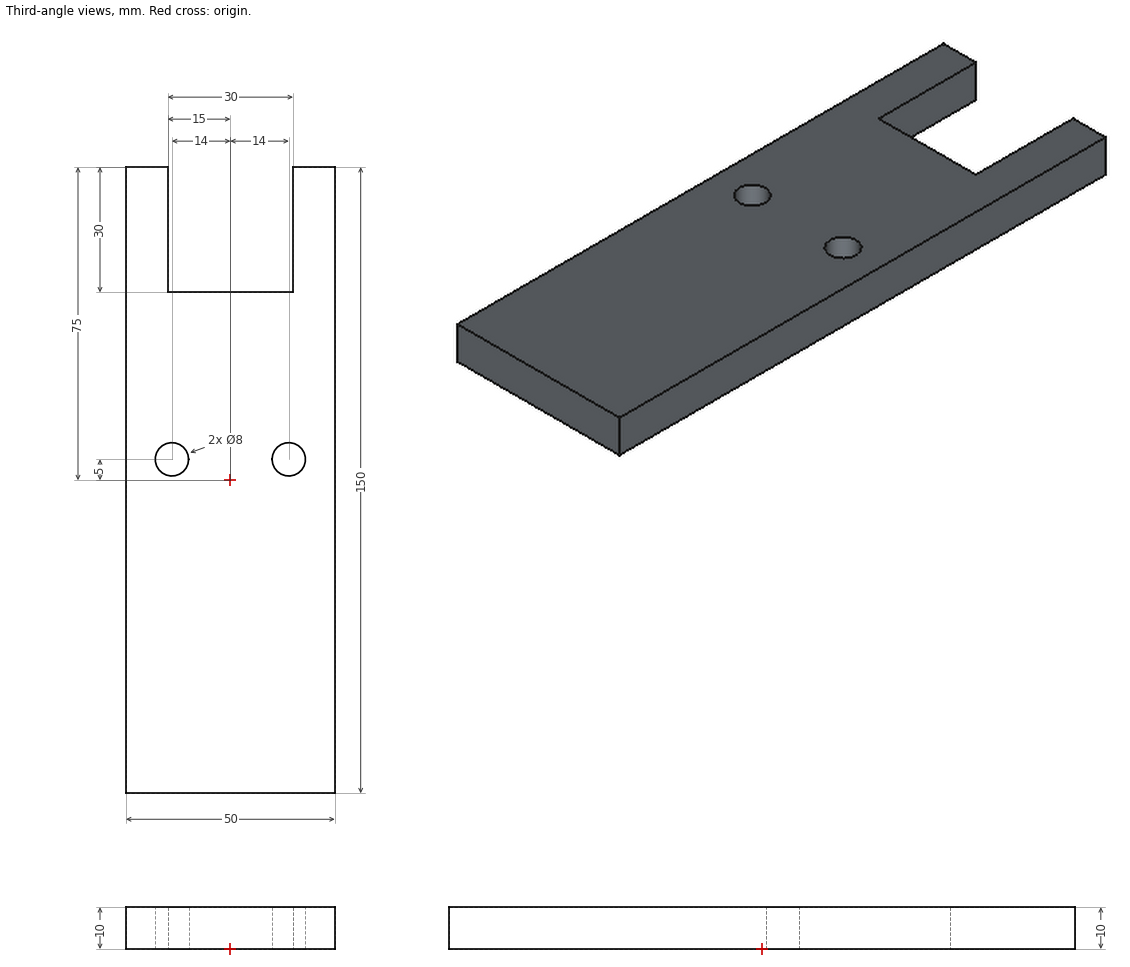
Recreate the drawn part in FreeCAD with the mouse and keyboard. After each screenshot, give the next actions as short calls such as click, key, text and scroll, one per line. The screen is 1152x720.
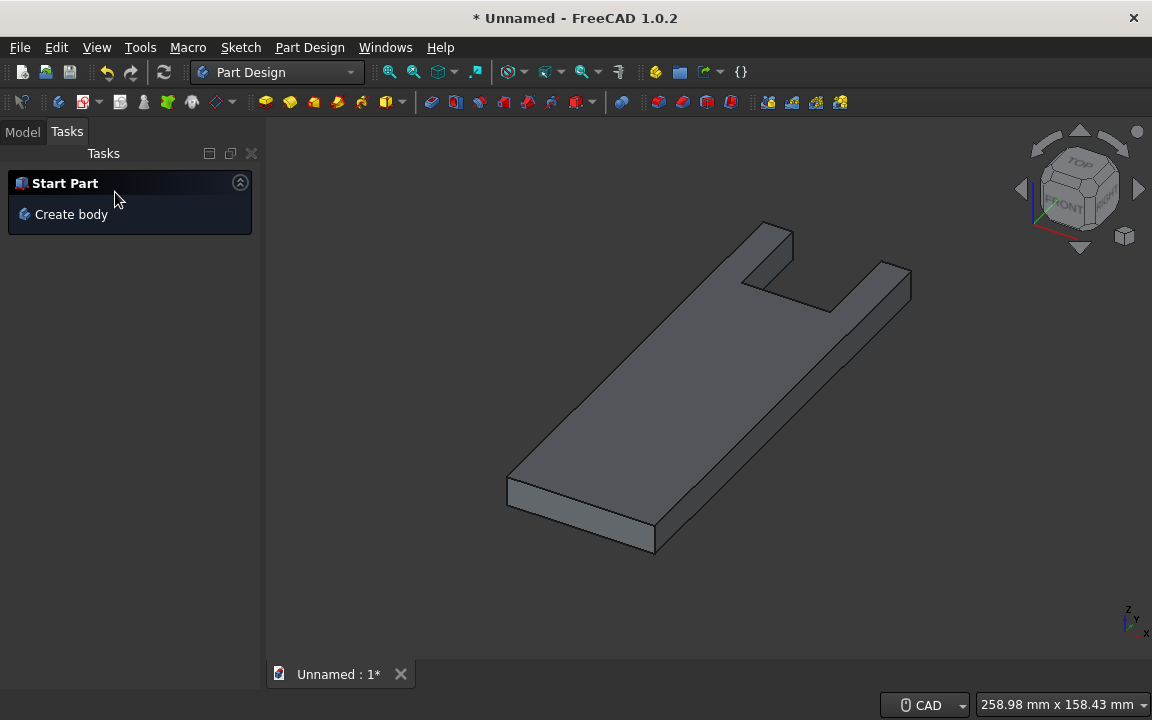
click(709, 373)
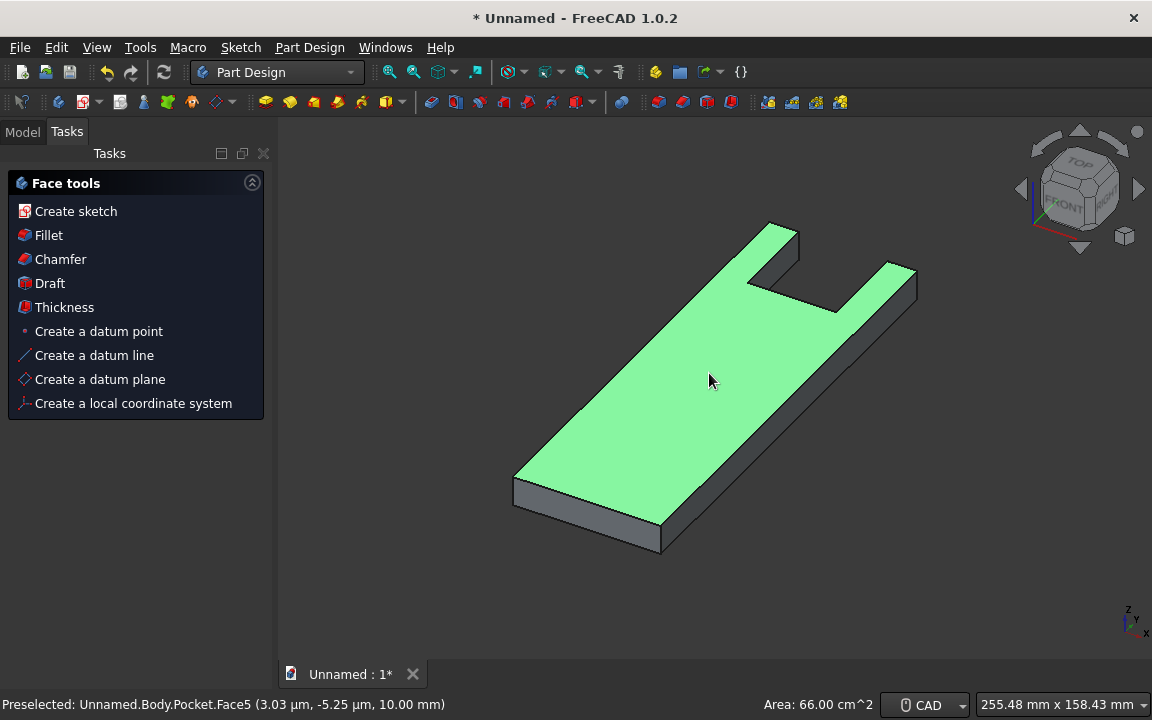
click(84, 102)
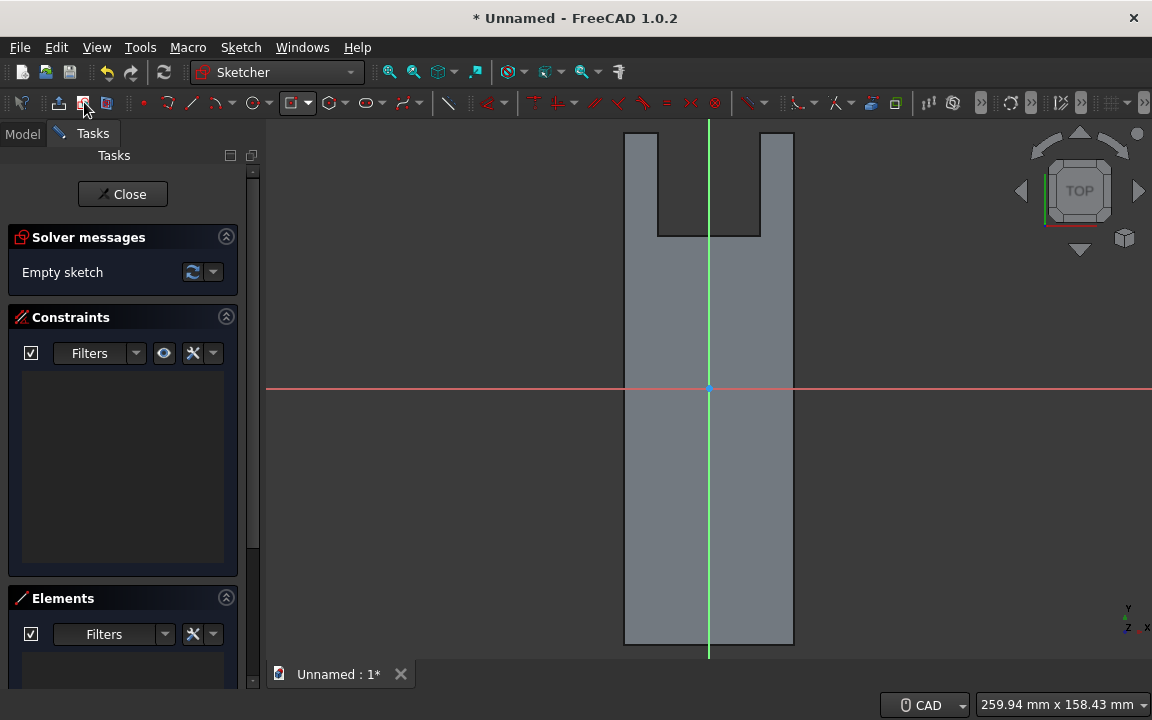
scroll(731, 369, up, 7)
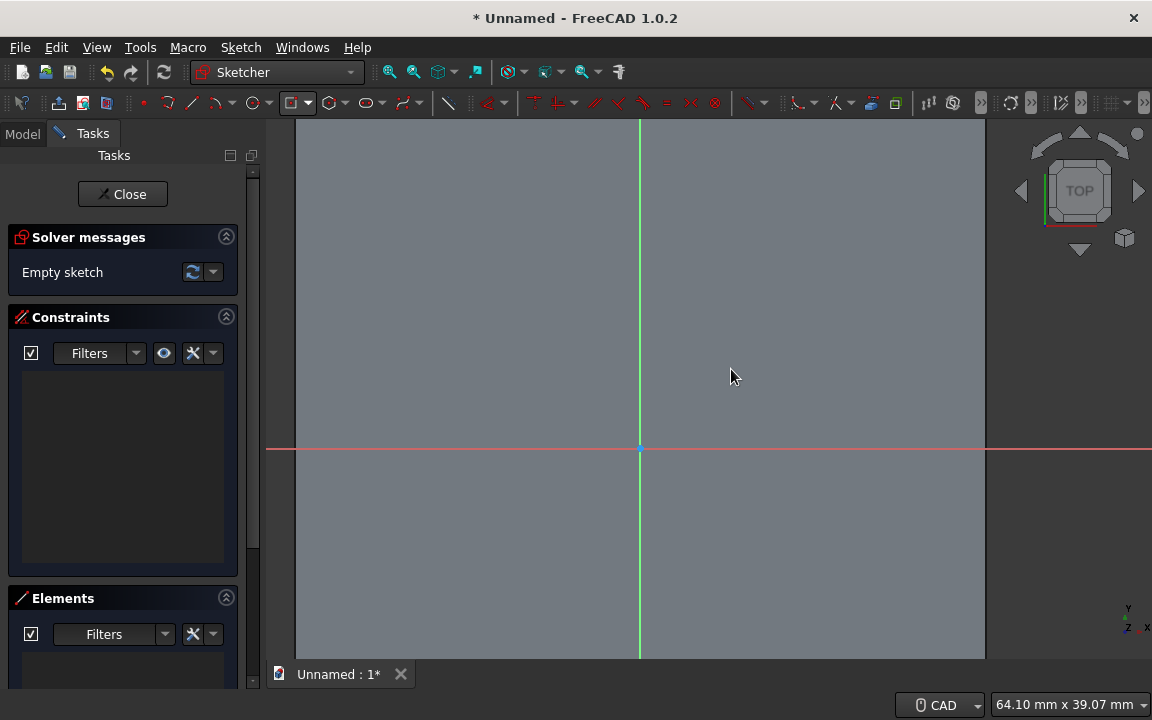
key(g)
key(c)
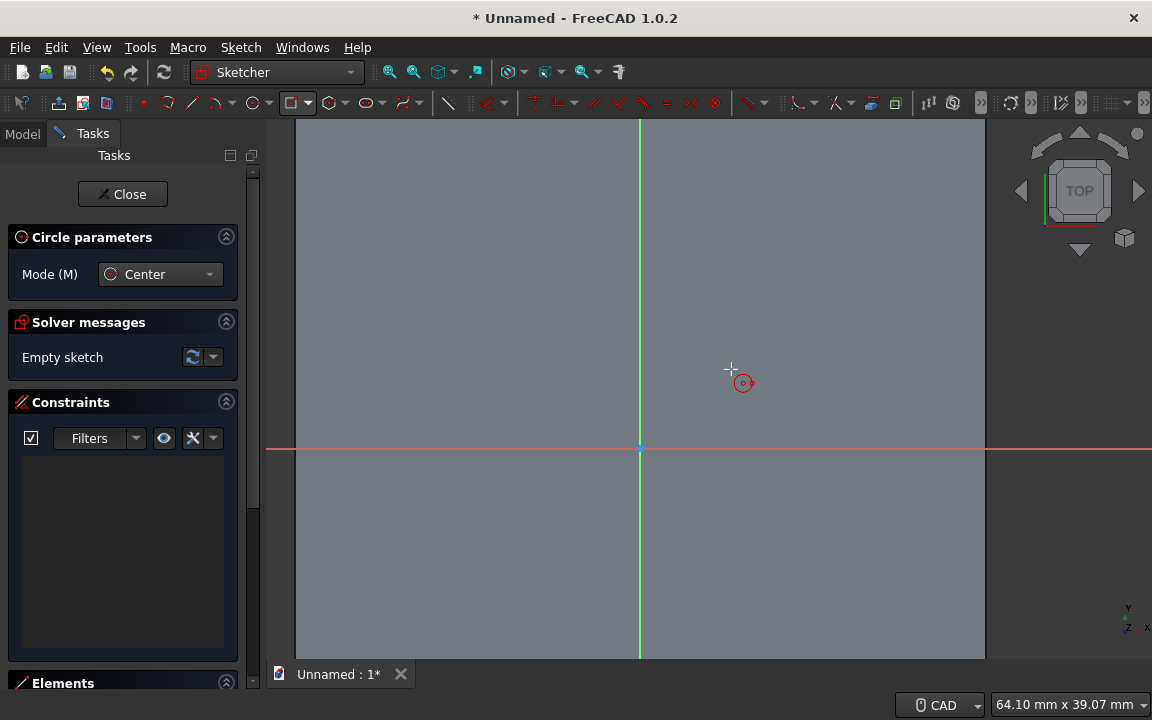
click(447, 380)
click(486, 340)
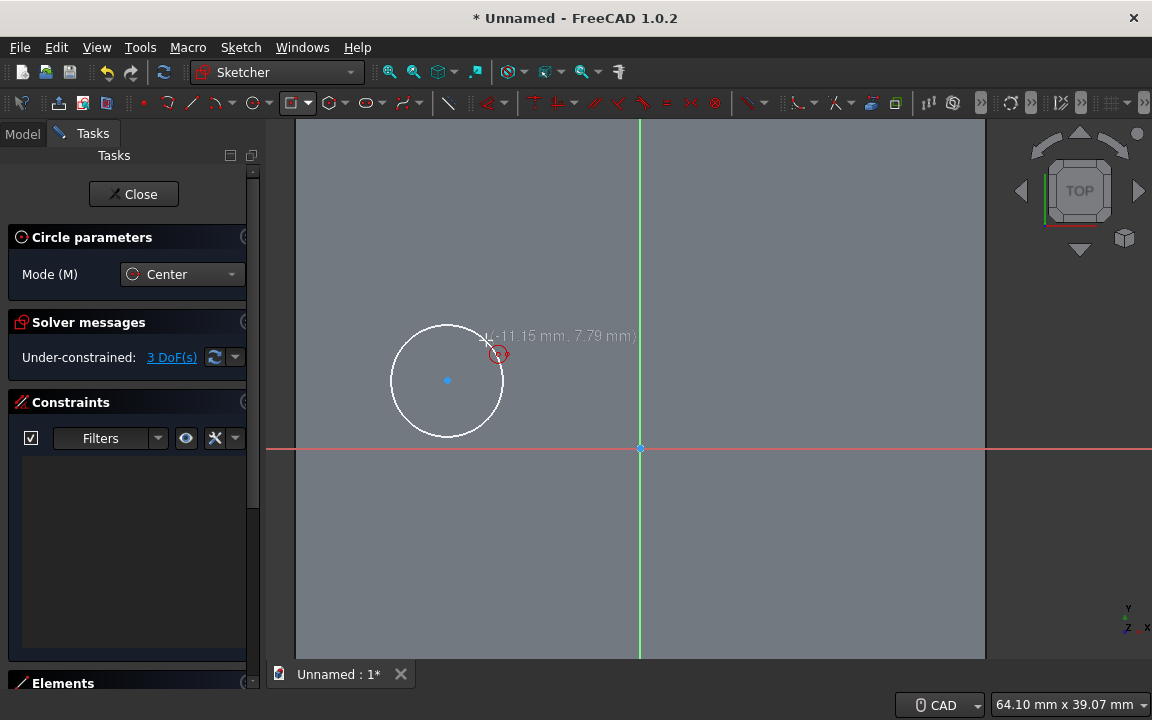
click(834, 380)
click(873, 340)
key(Escape)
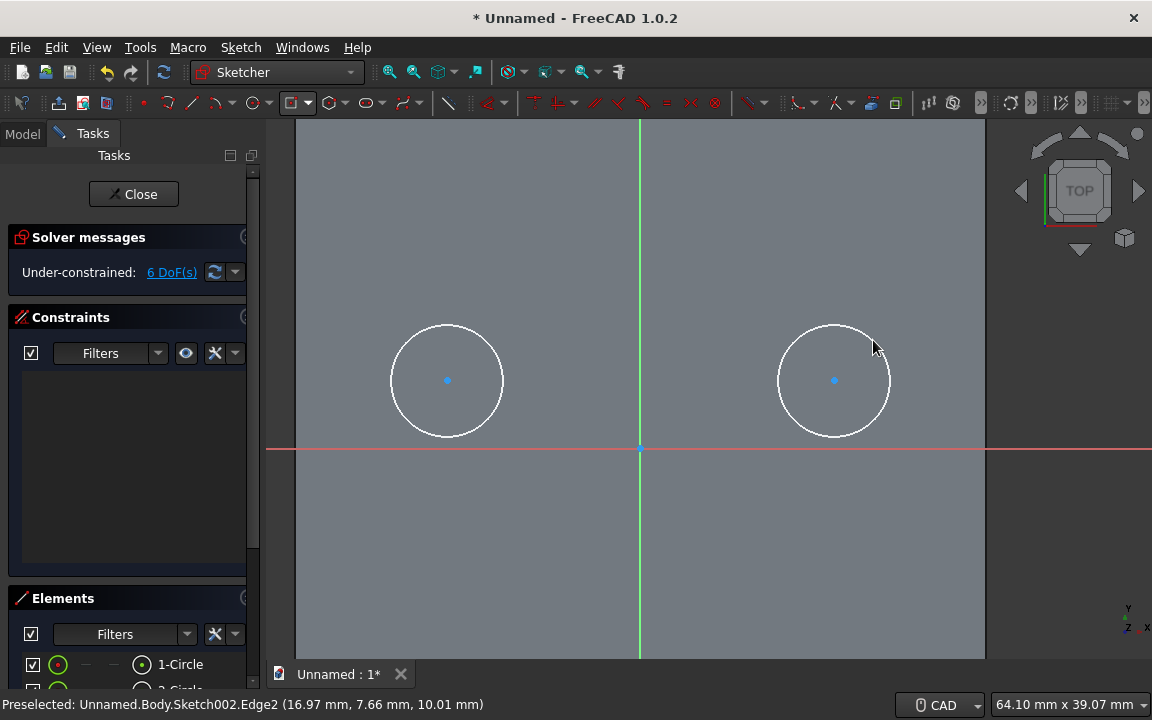
click(486, 341)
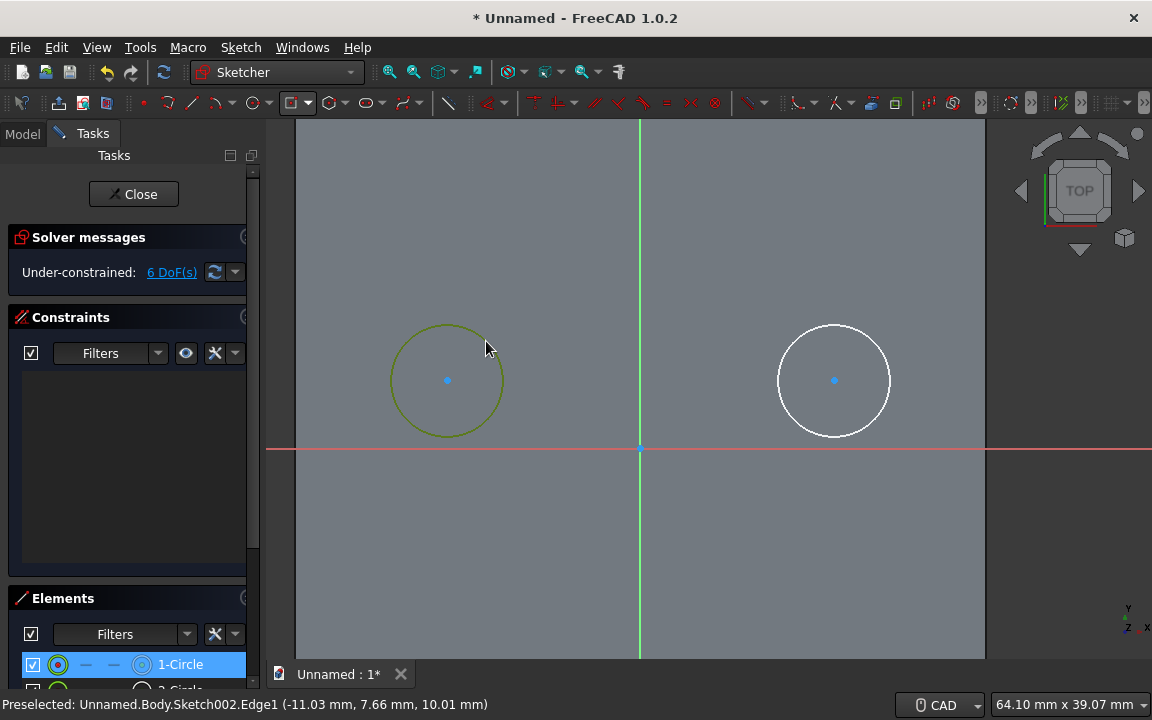
click(873, 341)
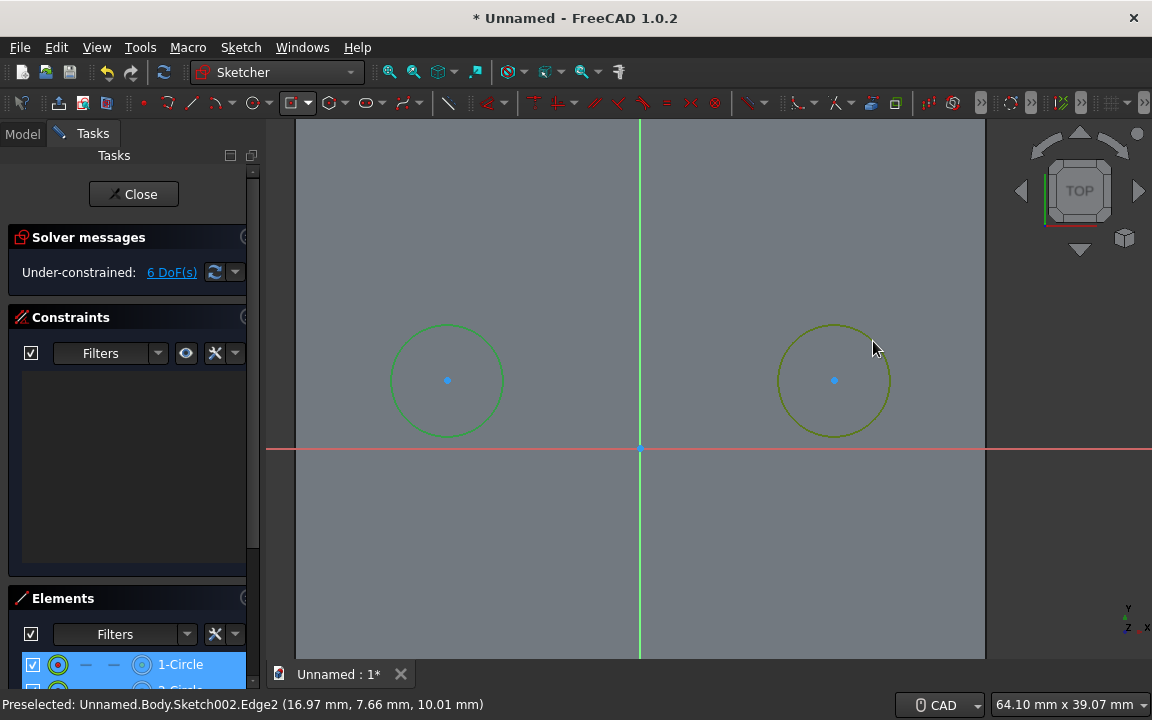
key(e)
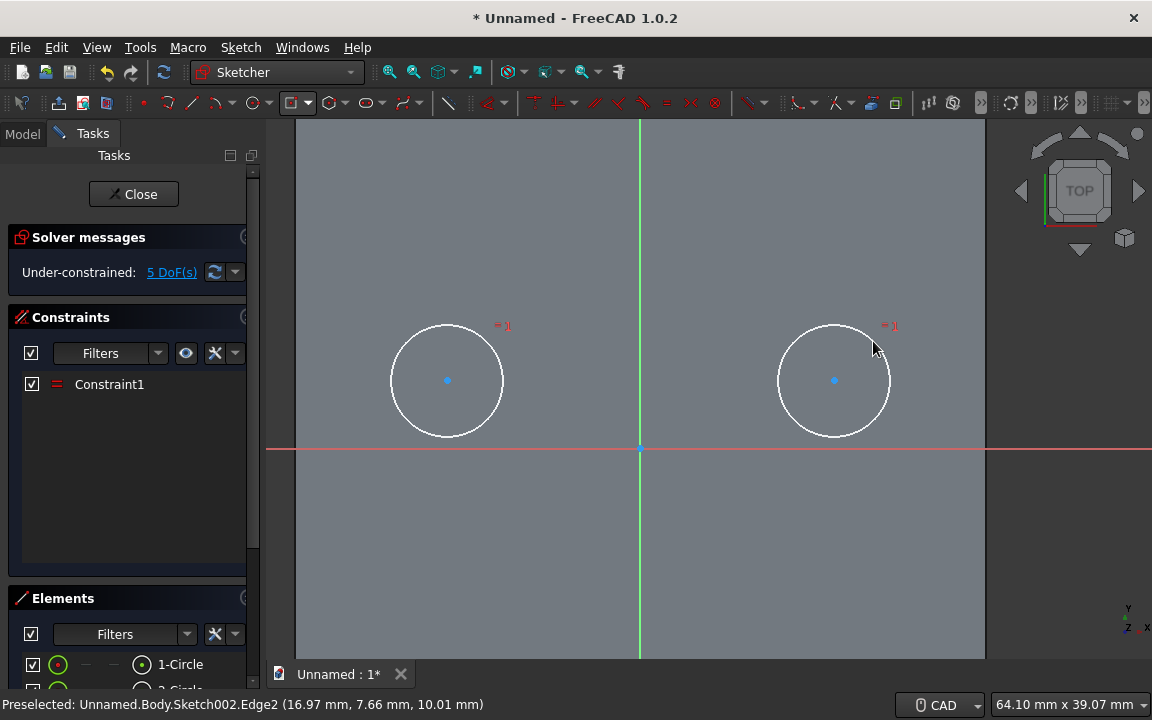
click(447, 381)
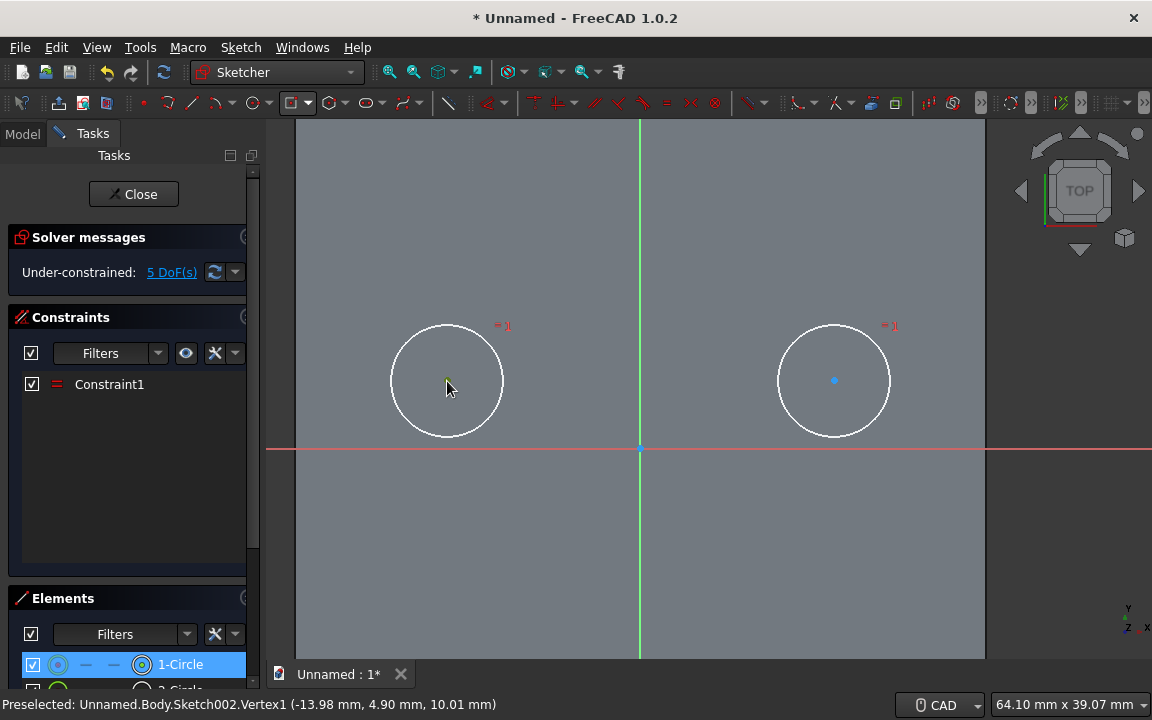
click(834, 381)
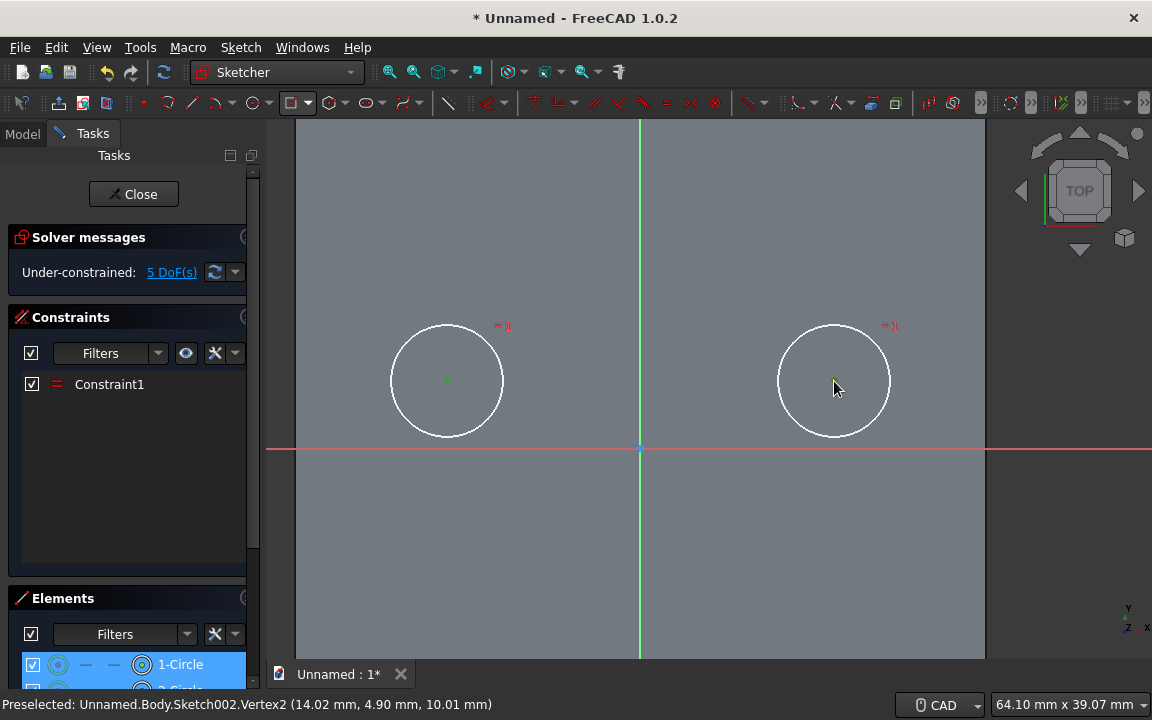
key(h)